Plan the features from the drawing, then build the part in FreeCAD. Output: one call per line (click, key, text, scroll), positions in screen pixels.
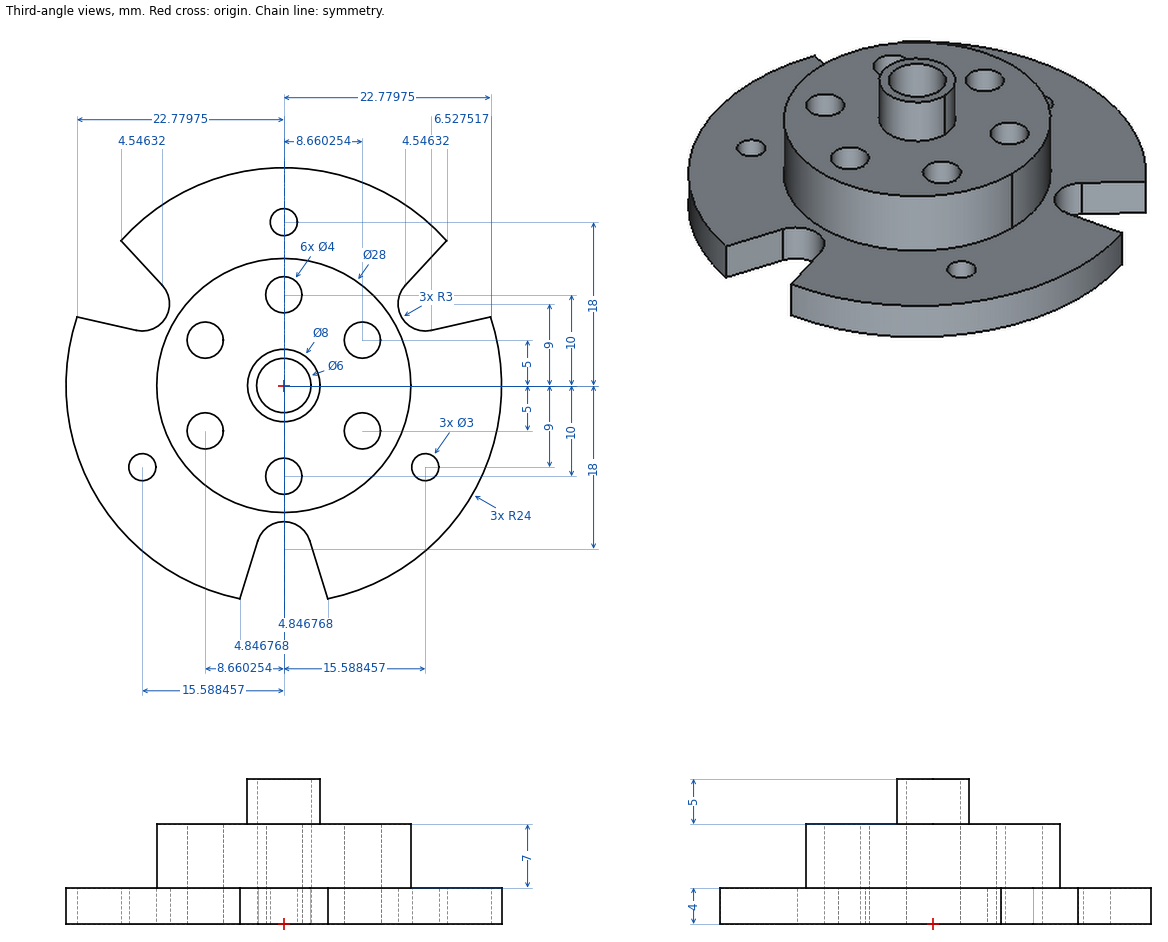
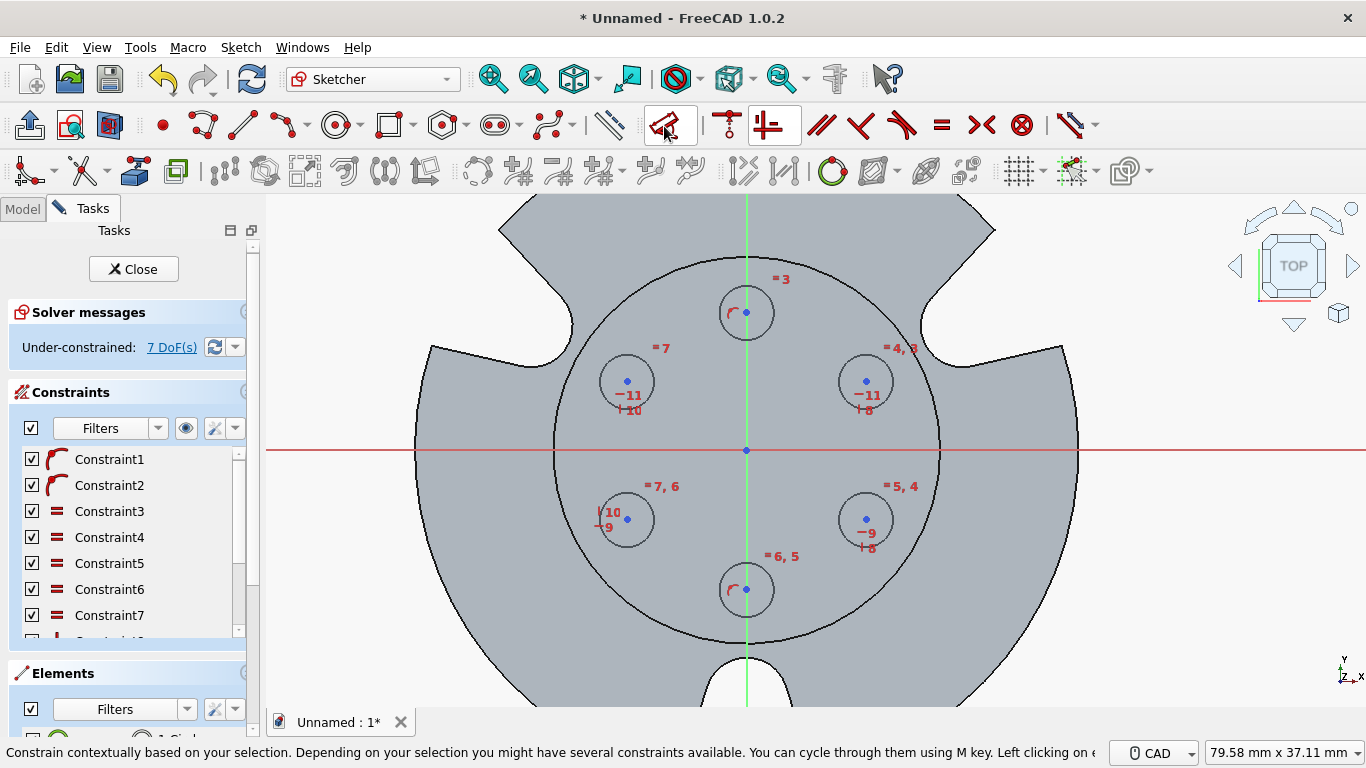
click(766, 294)
click(789, 272)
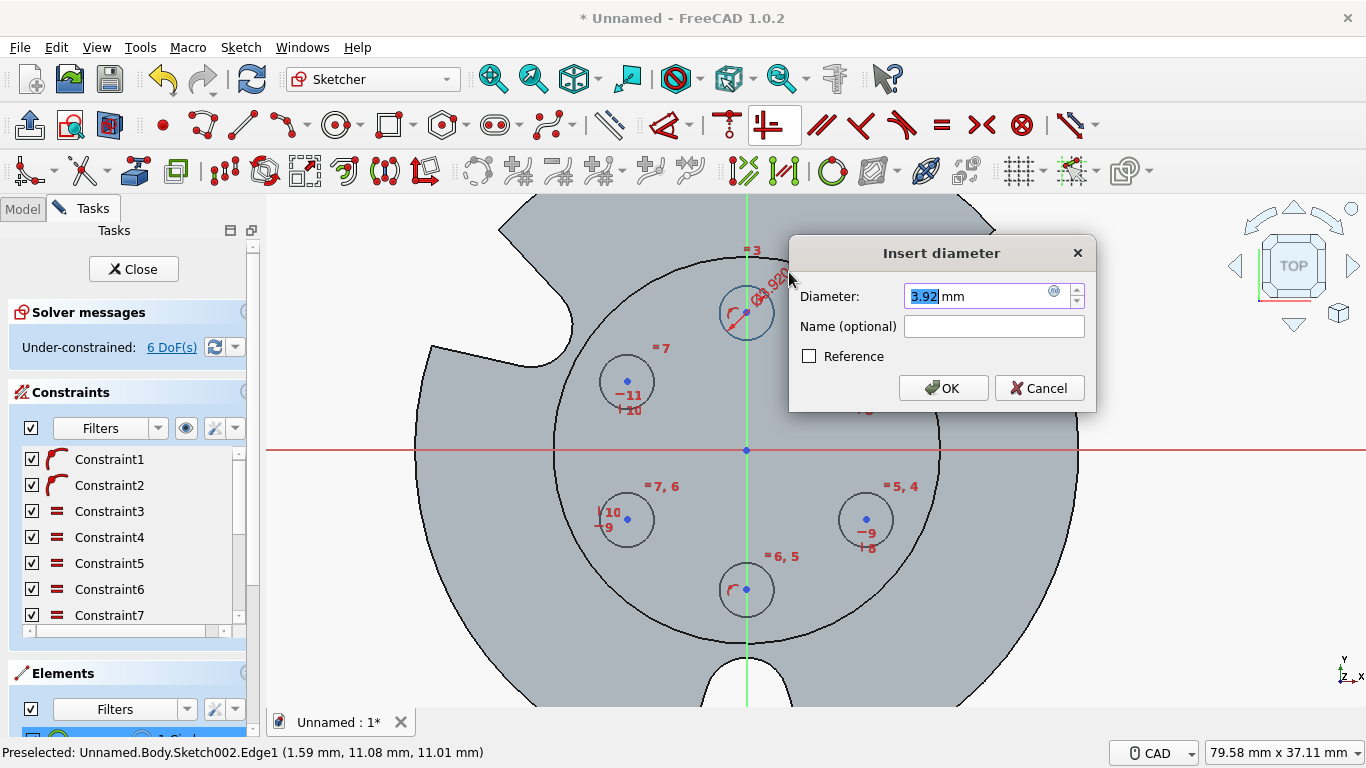
text(4)
key(Return)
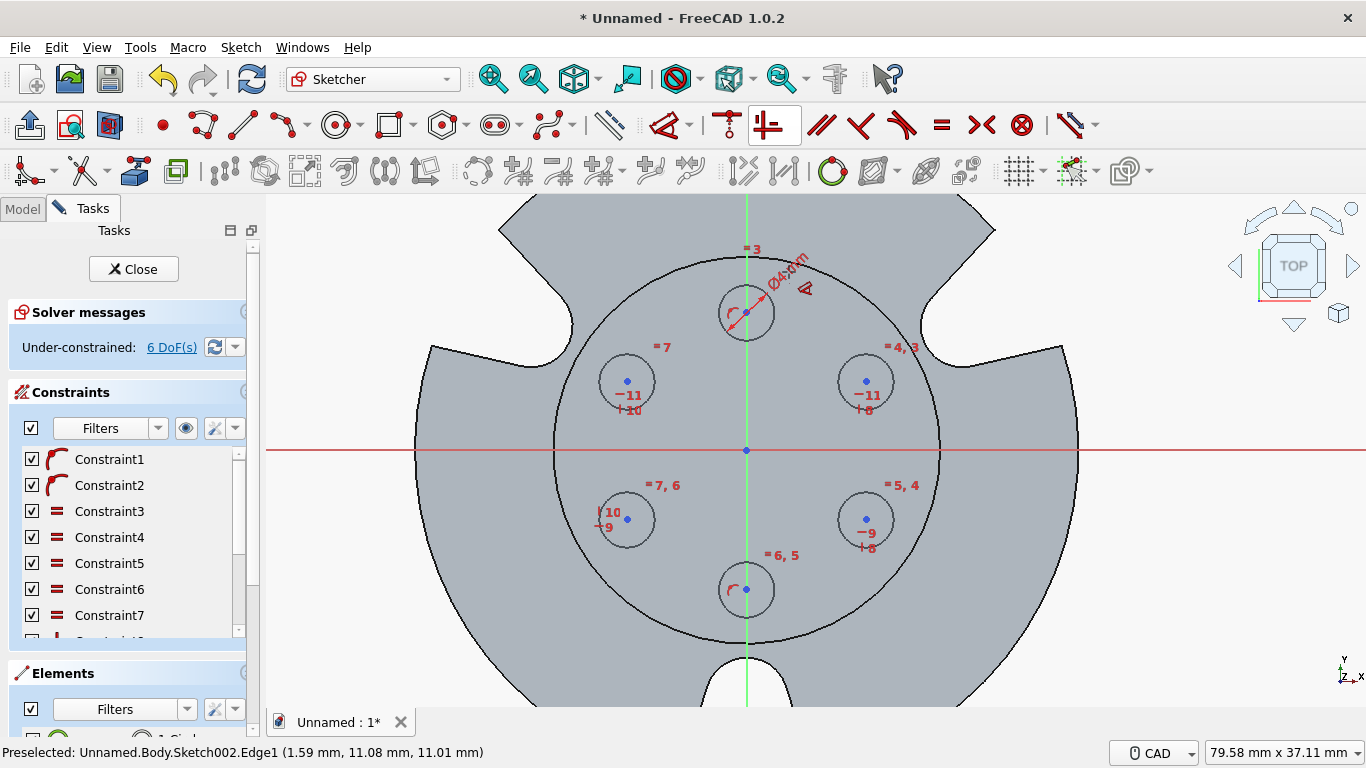
click(866, 382)
click(900, 416)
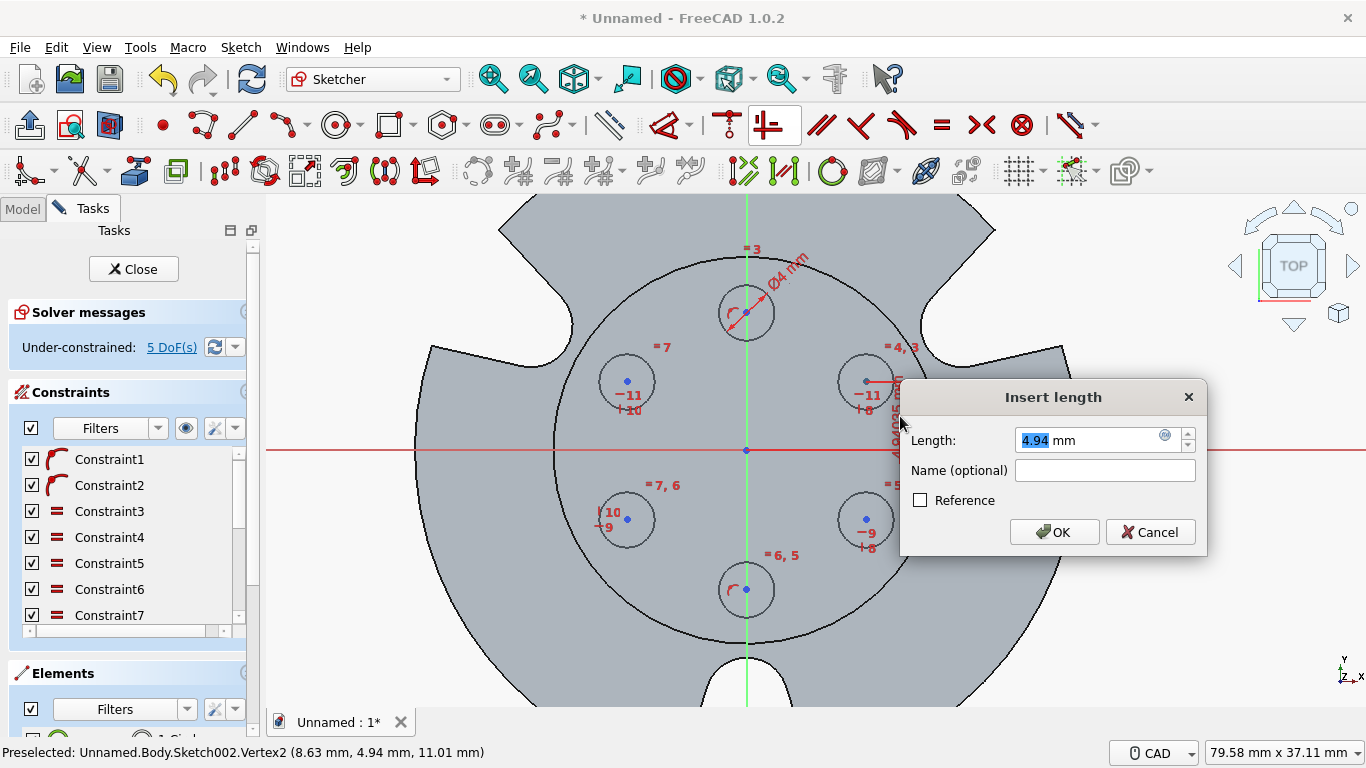
text(5)
key(Return)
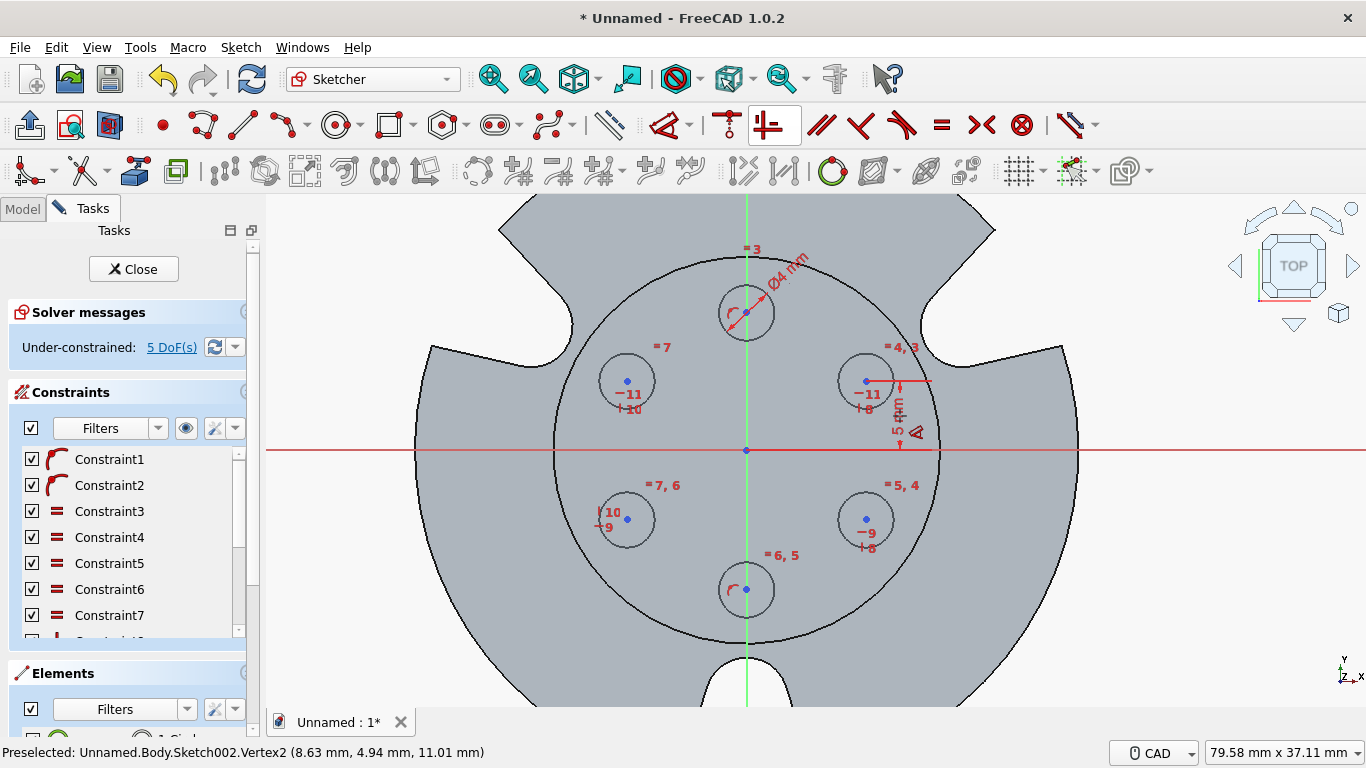
click(866, 520)
click(900, 485)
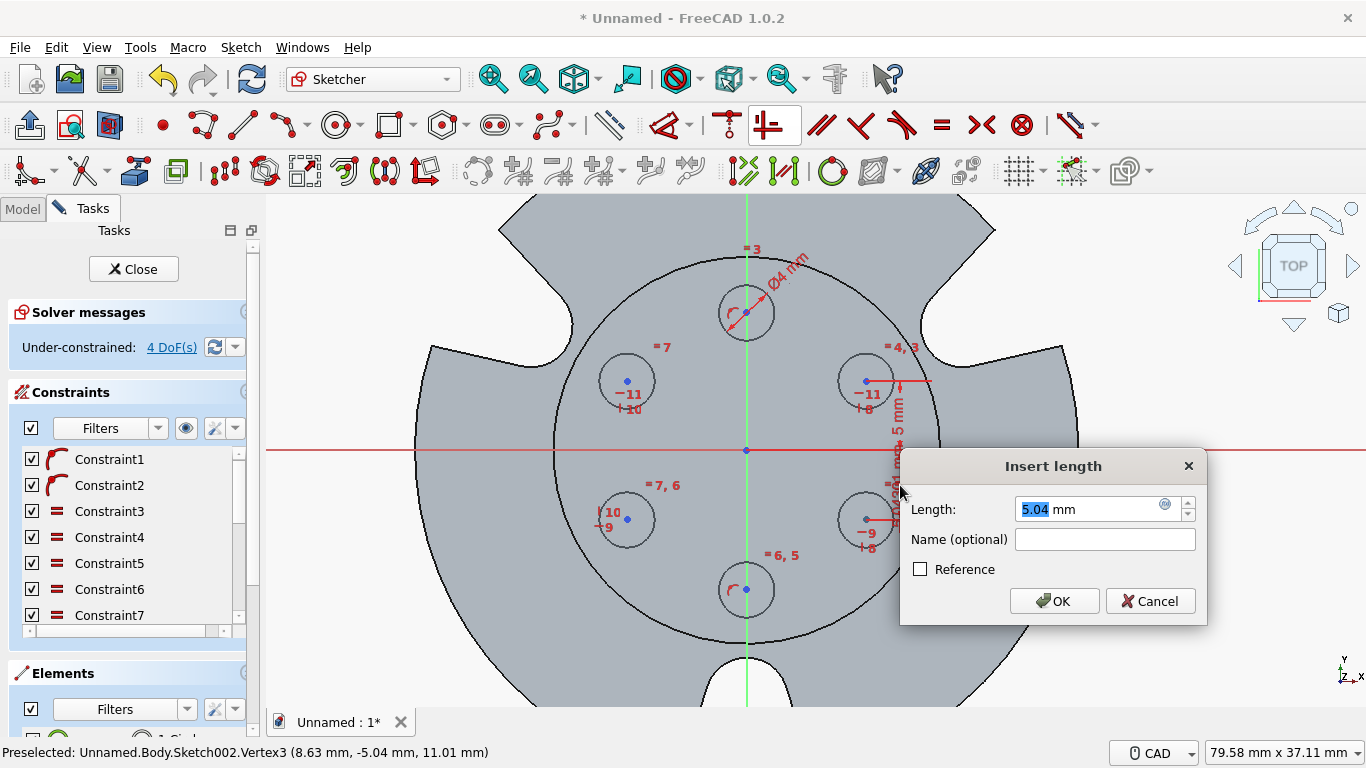
text(5)
key(Return)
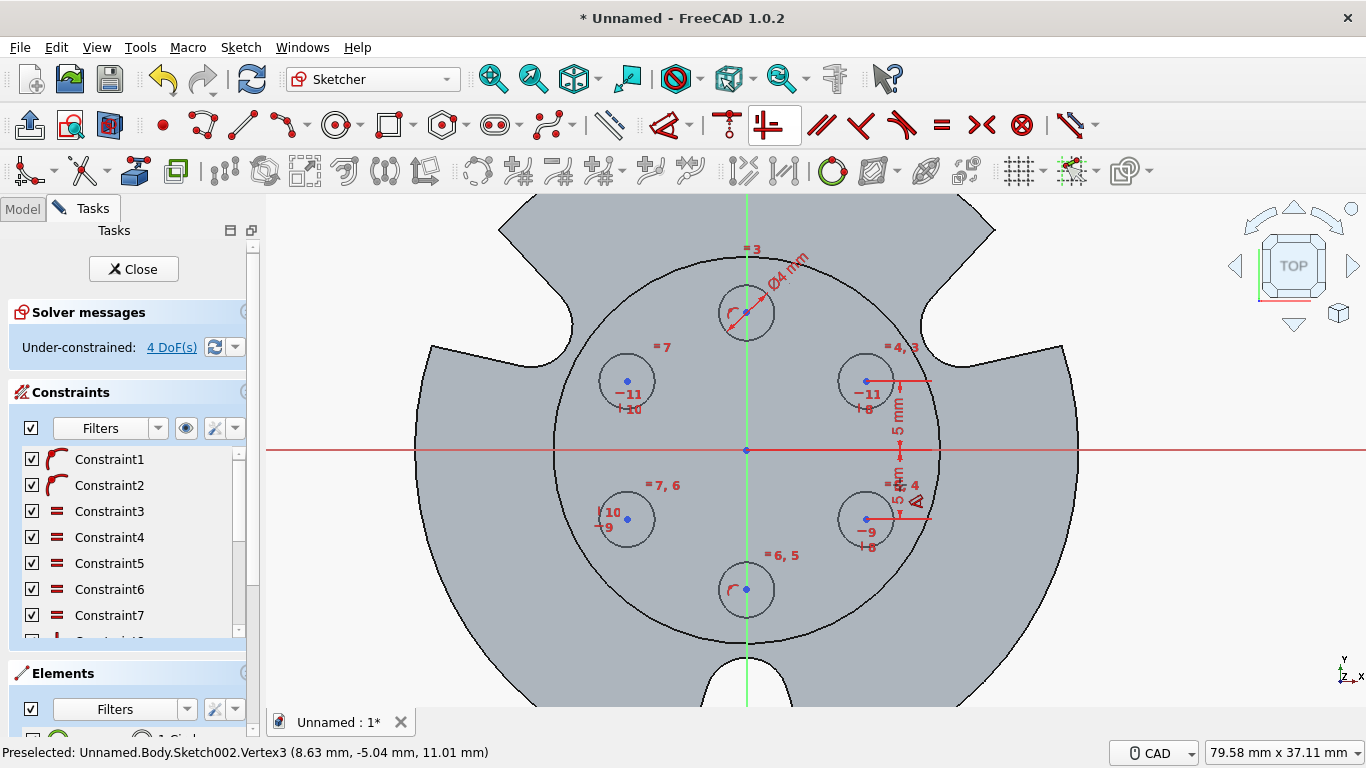
click(747, 313)
click(781, 382)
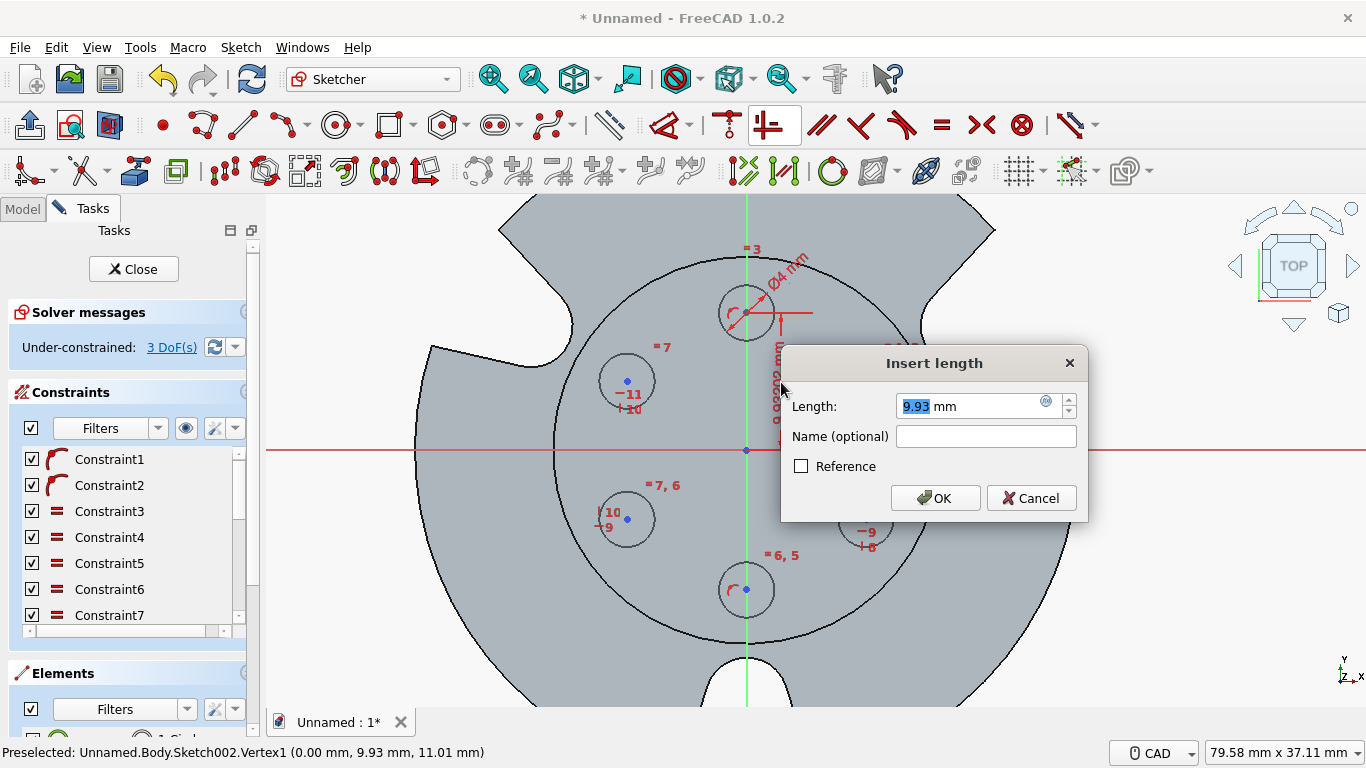
text(10)
key(Return)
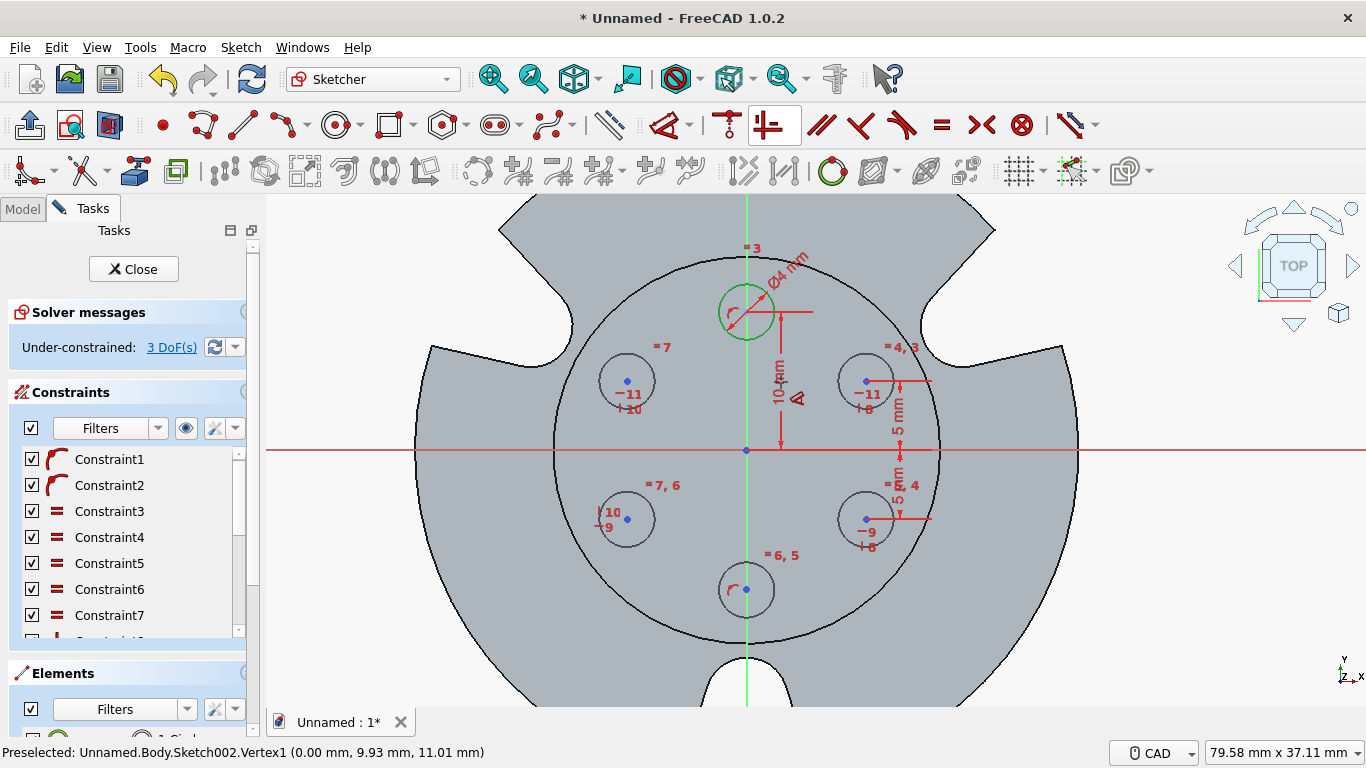
click(747, 590)
click(781, 520)